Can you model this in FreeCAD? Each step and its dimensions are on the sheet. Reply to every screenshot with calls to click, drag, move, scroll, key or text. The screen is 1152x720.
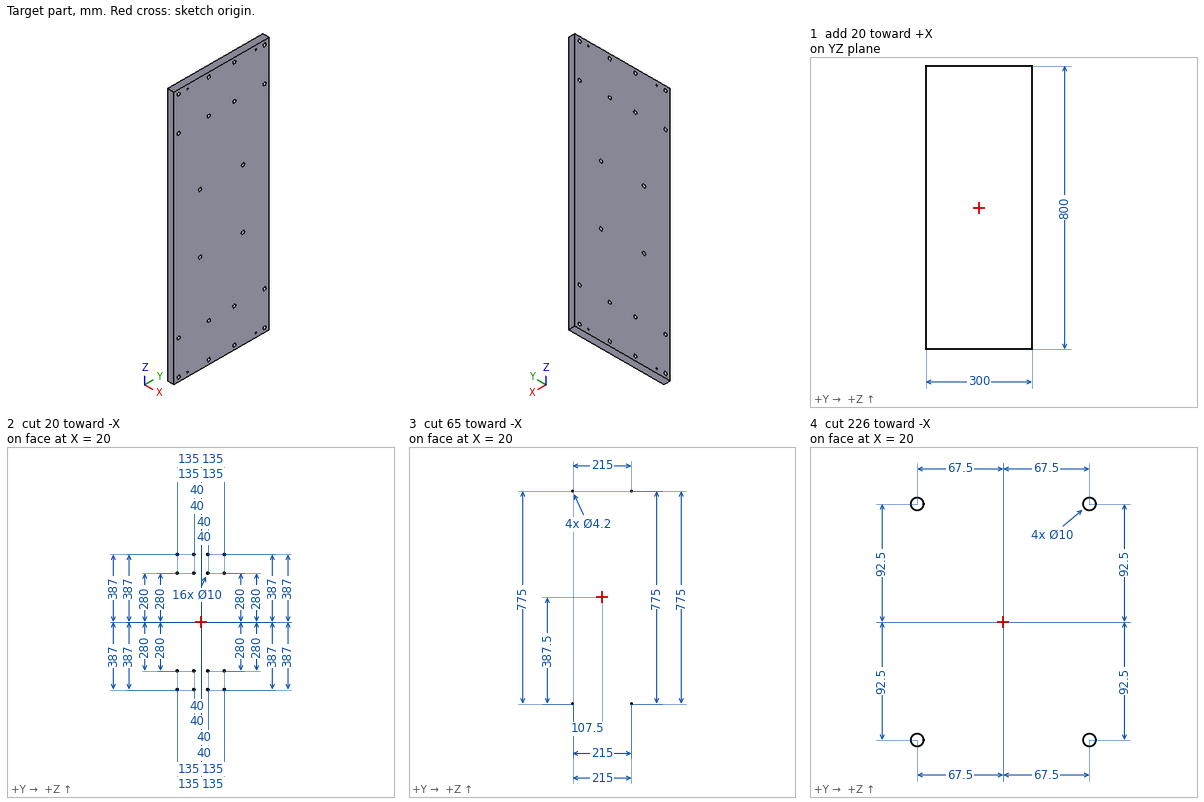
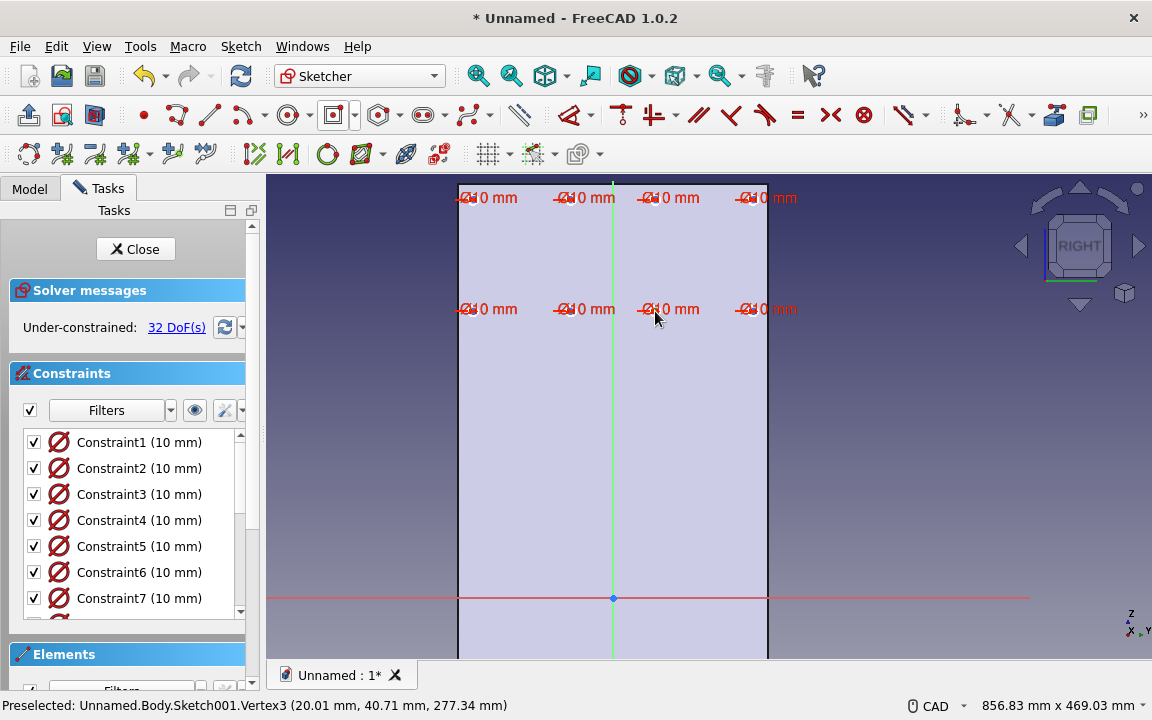
click(590, 116)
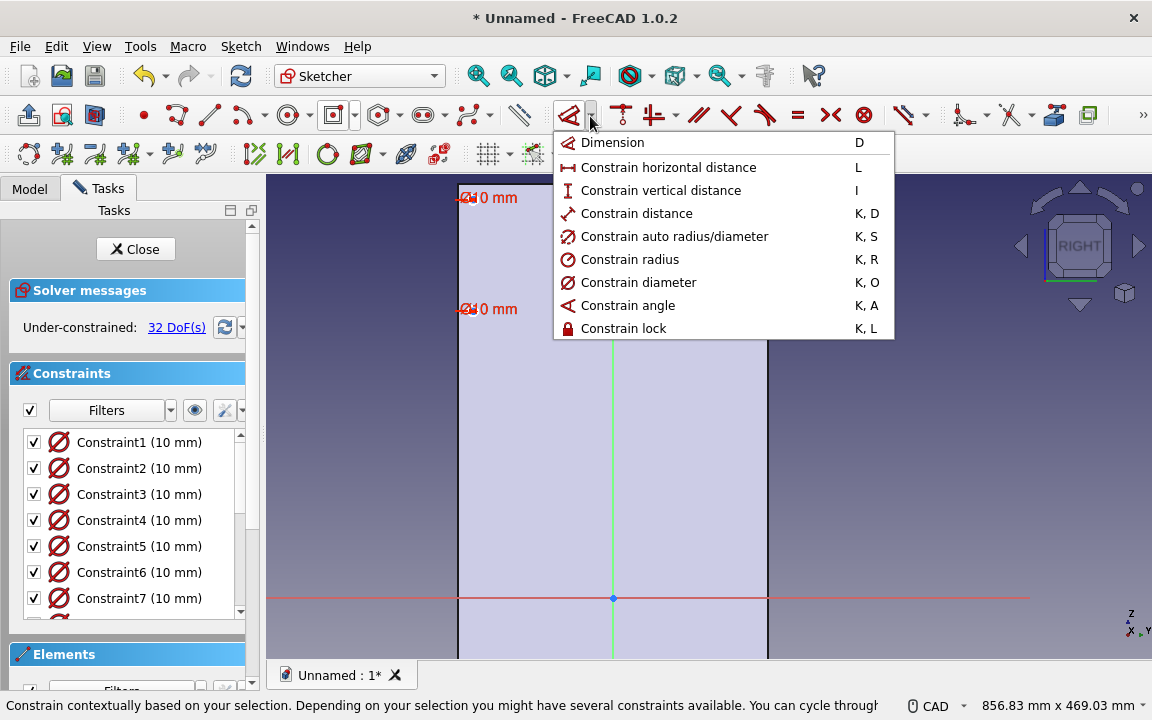
click(724, 168)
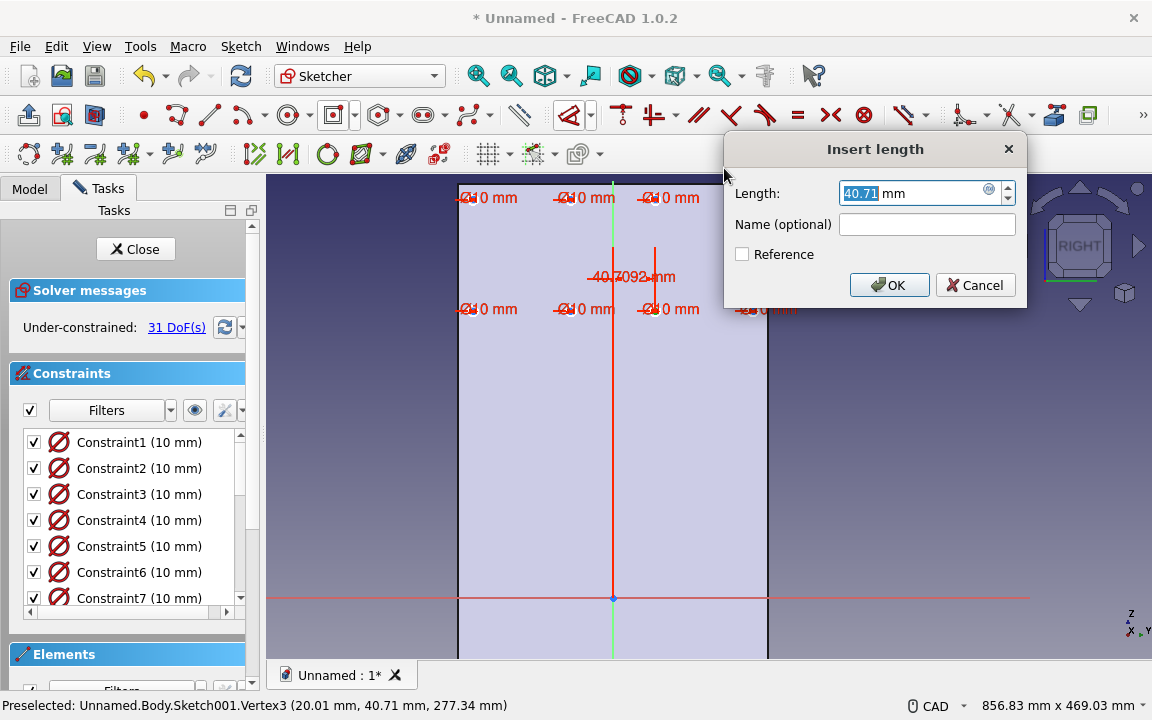
text(40)
key(Return)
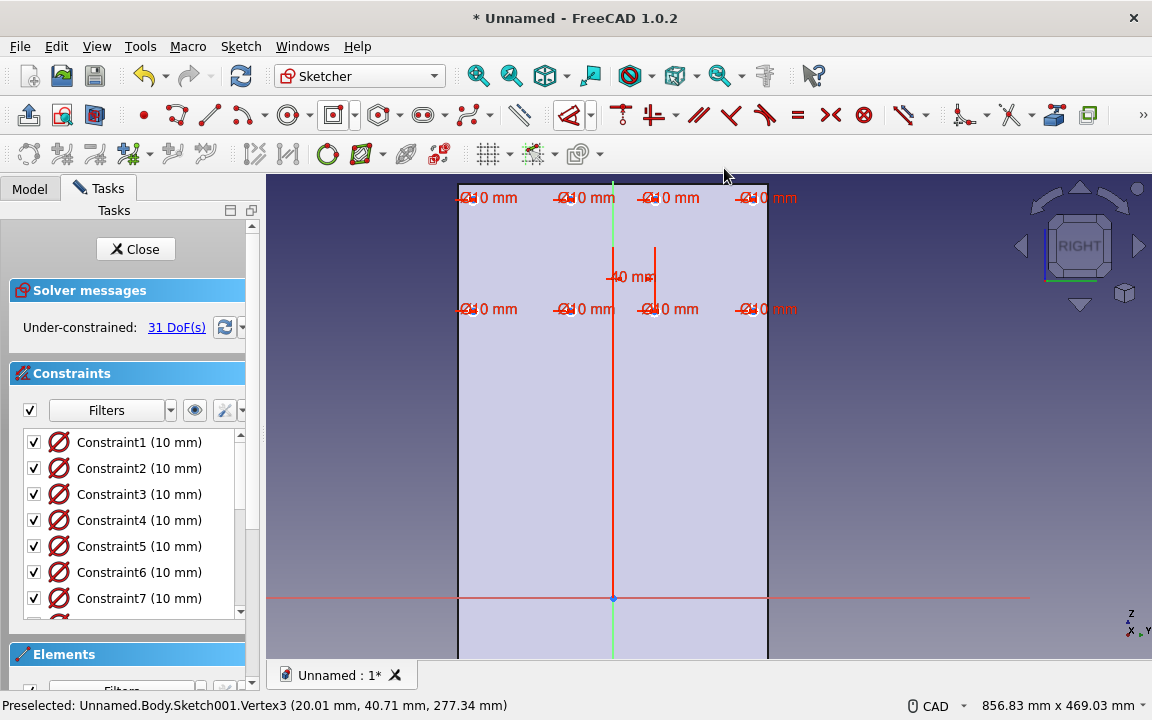
scroll(656, 311, down, 5)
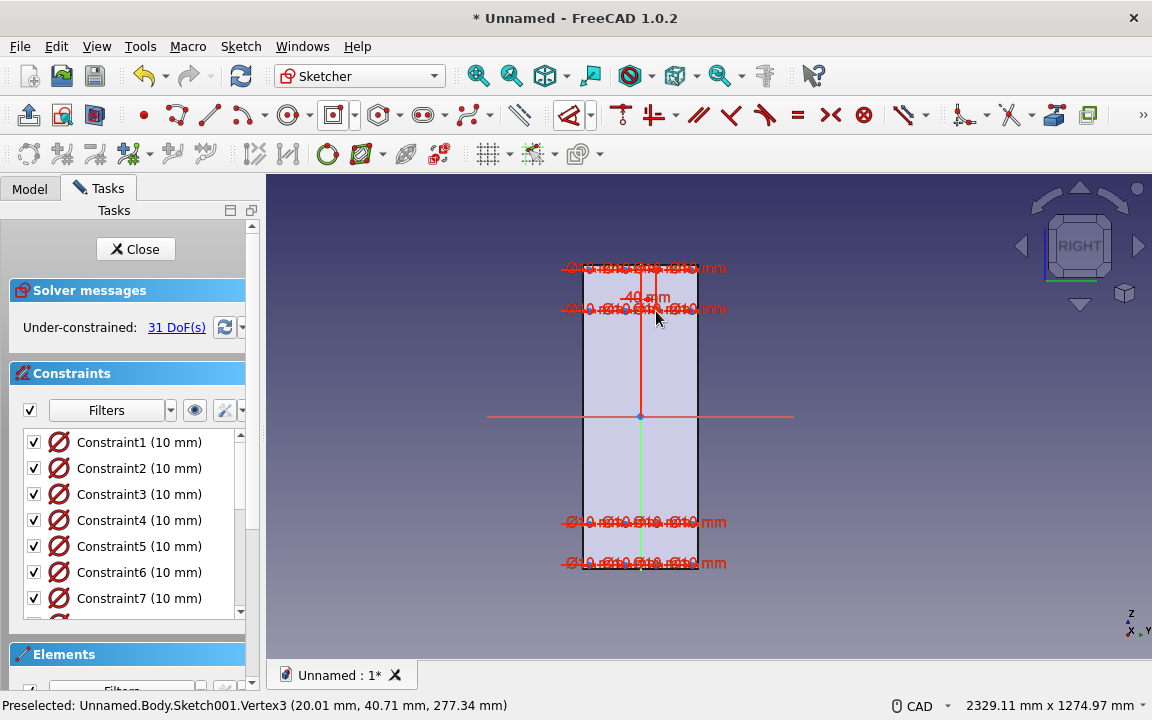
scroll(656, 270, up, 5)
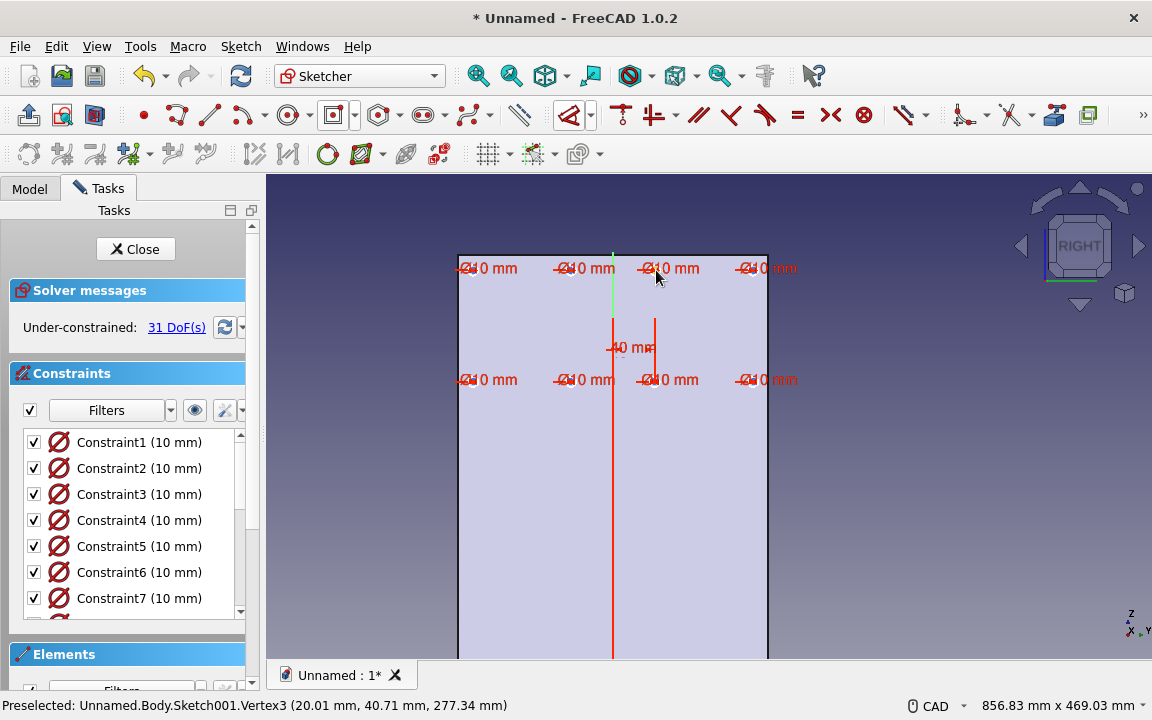
click(655, 270)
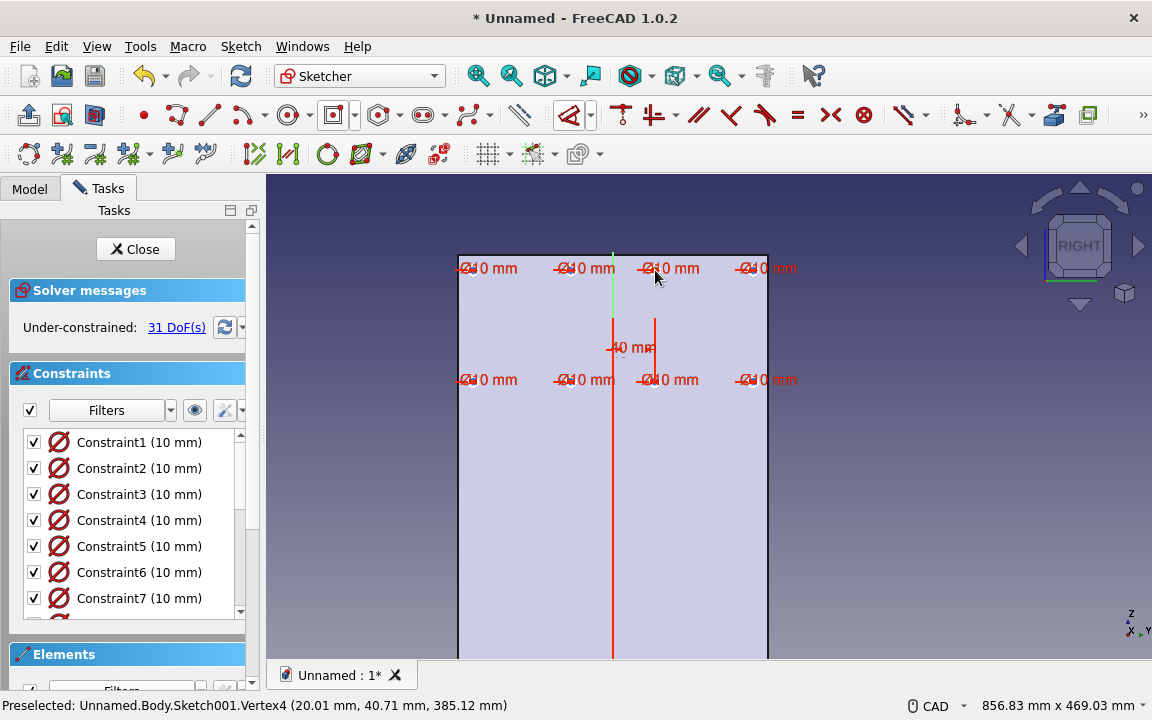
key(l)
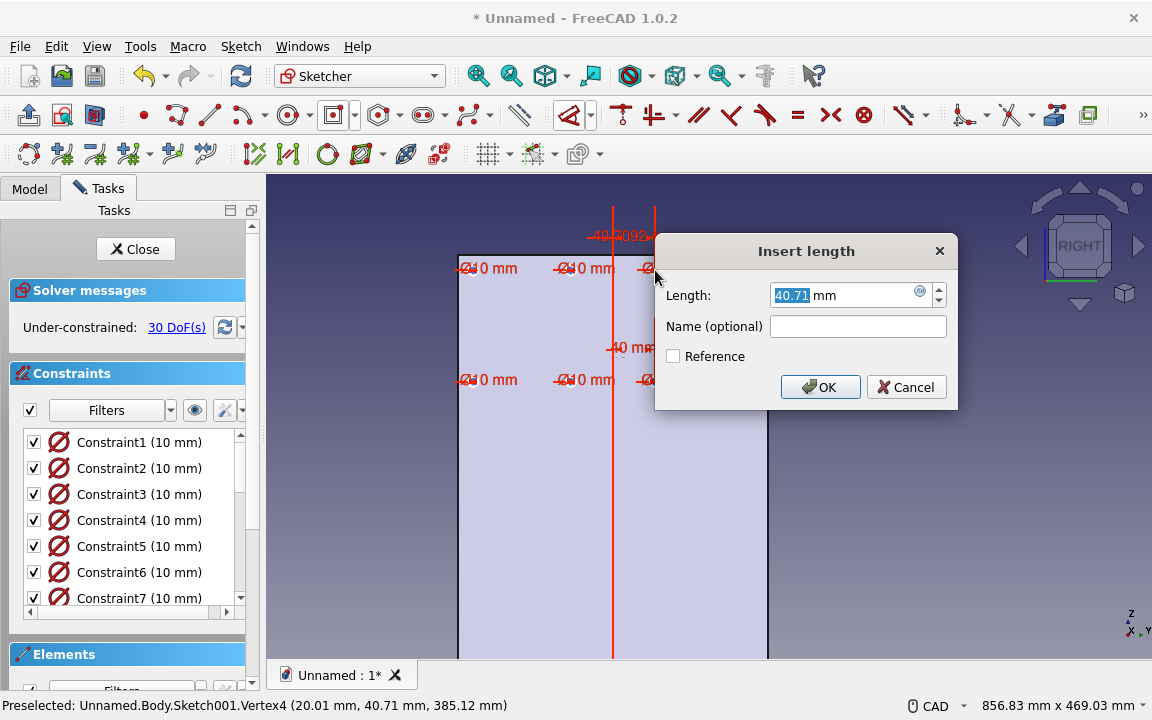
text(40)
key(Return)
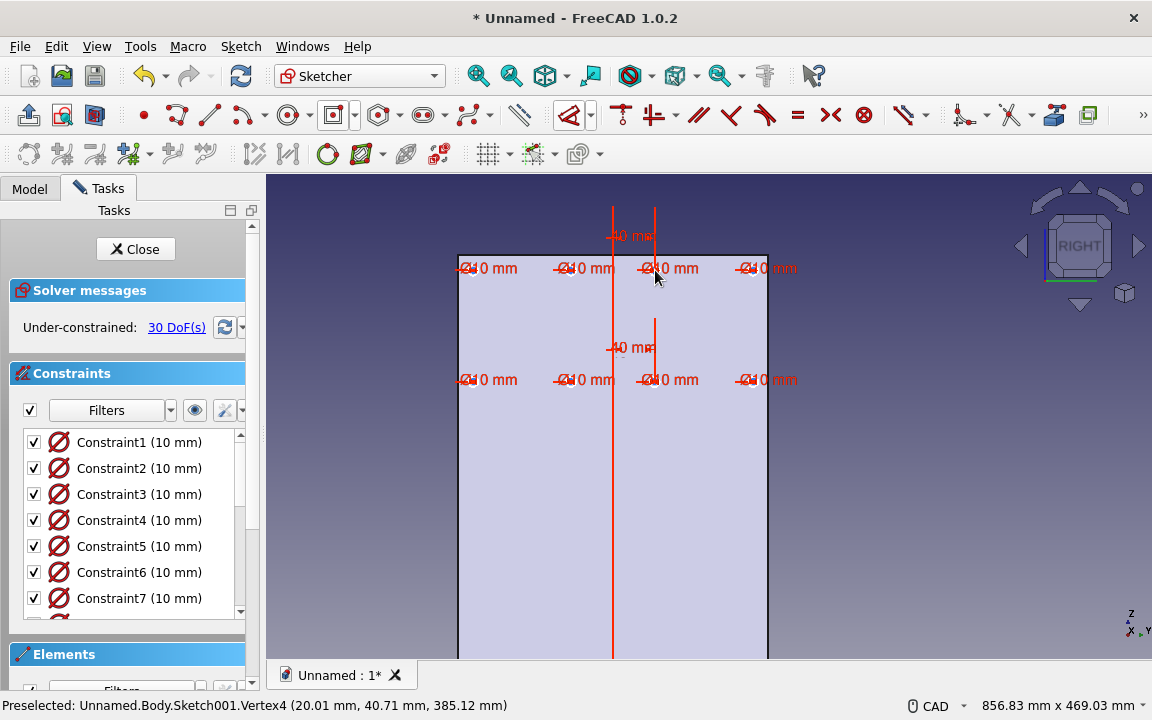
click(571, 382)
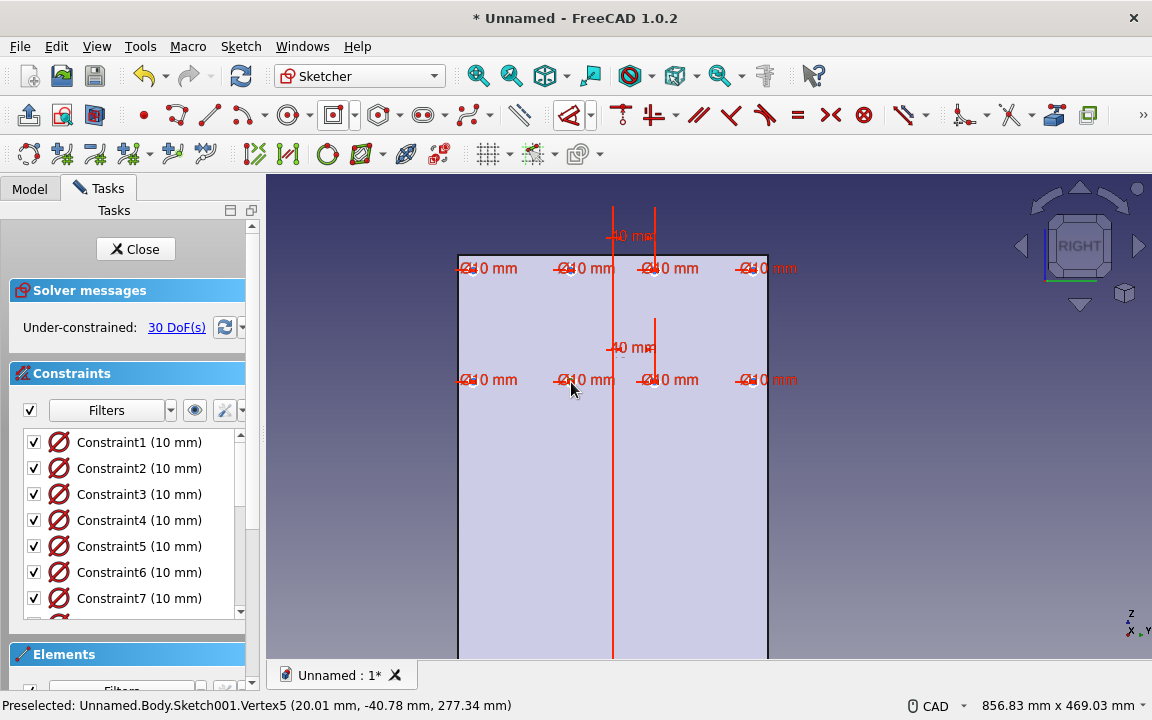
key(l)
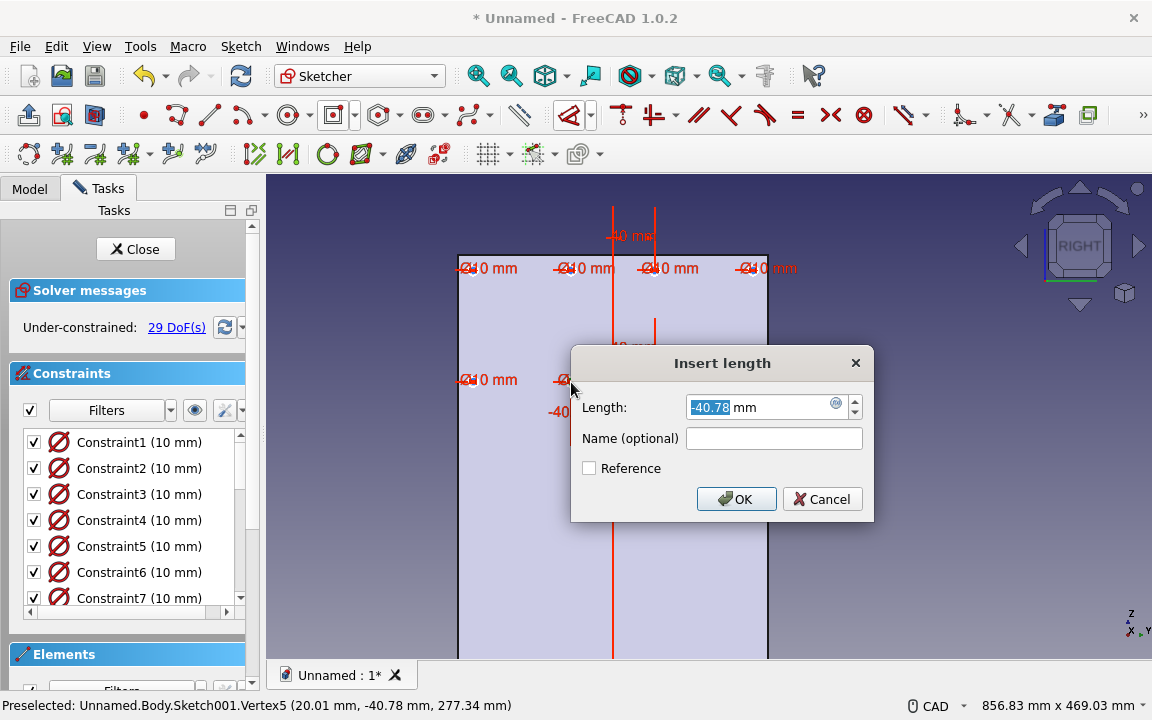
text(-40)
key(Return)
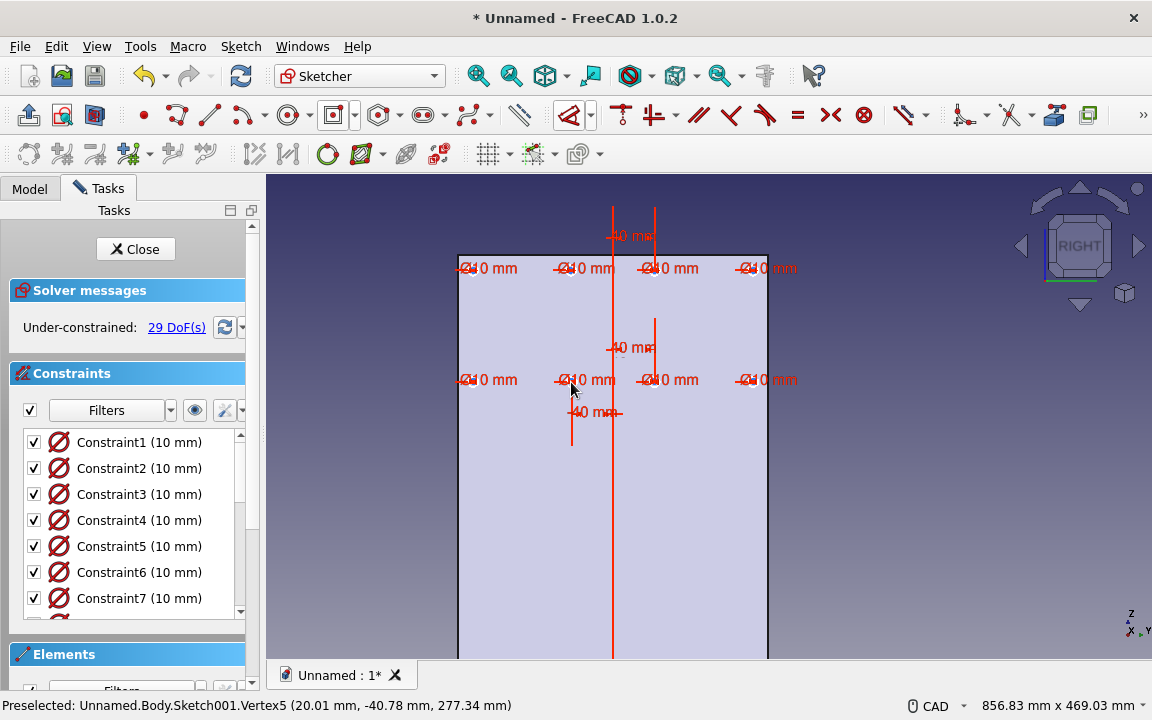
click(571, 270)